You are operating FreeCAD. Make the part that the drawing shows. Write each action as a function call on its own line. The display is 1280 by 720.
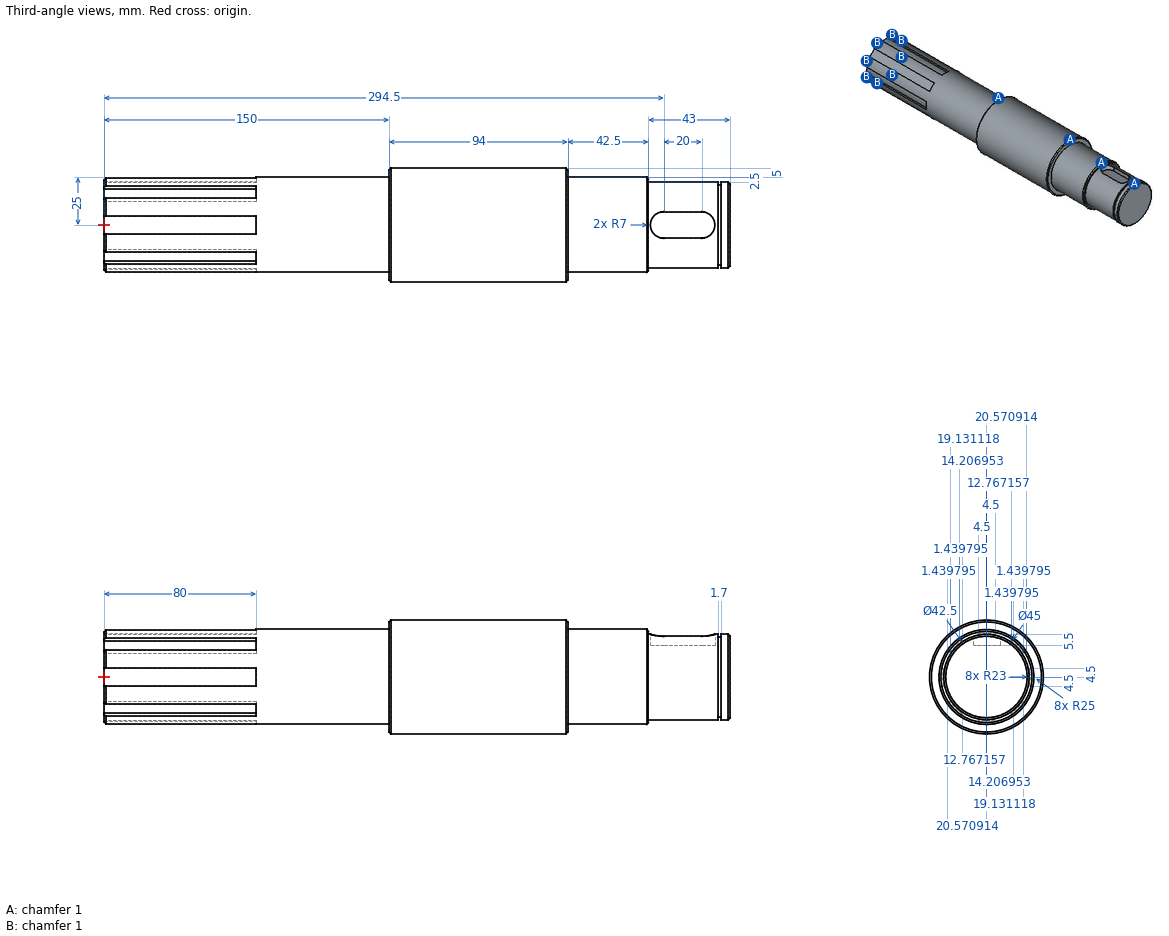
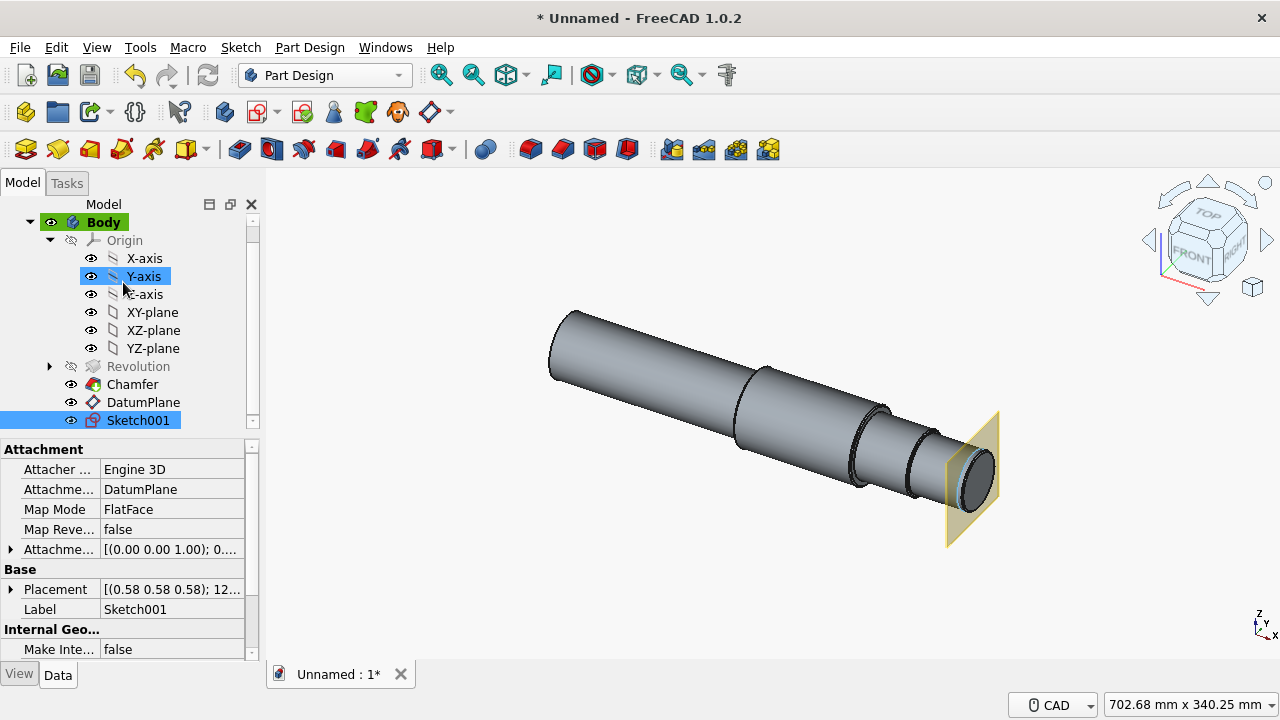
click(240, 150)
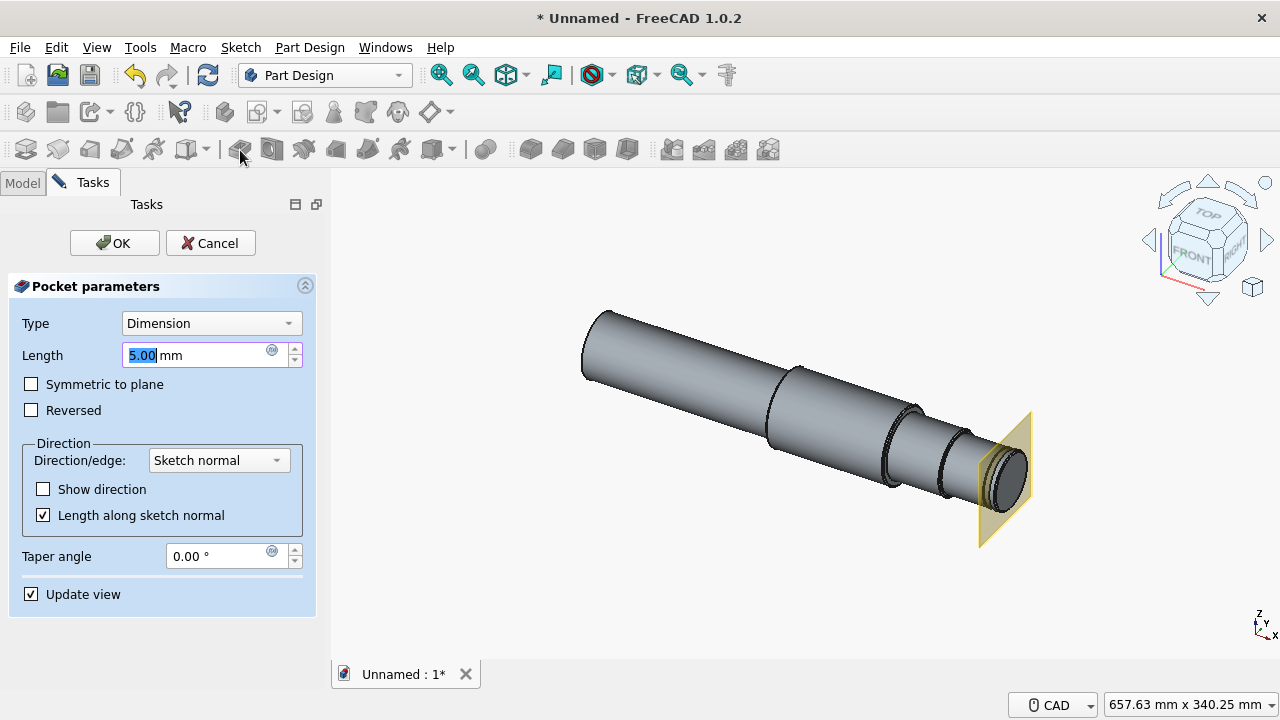
text(1.7)
key(Tab)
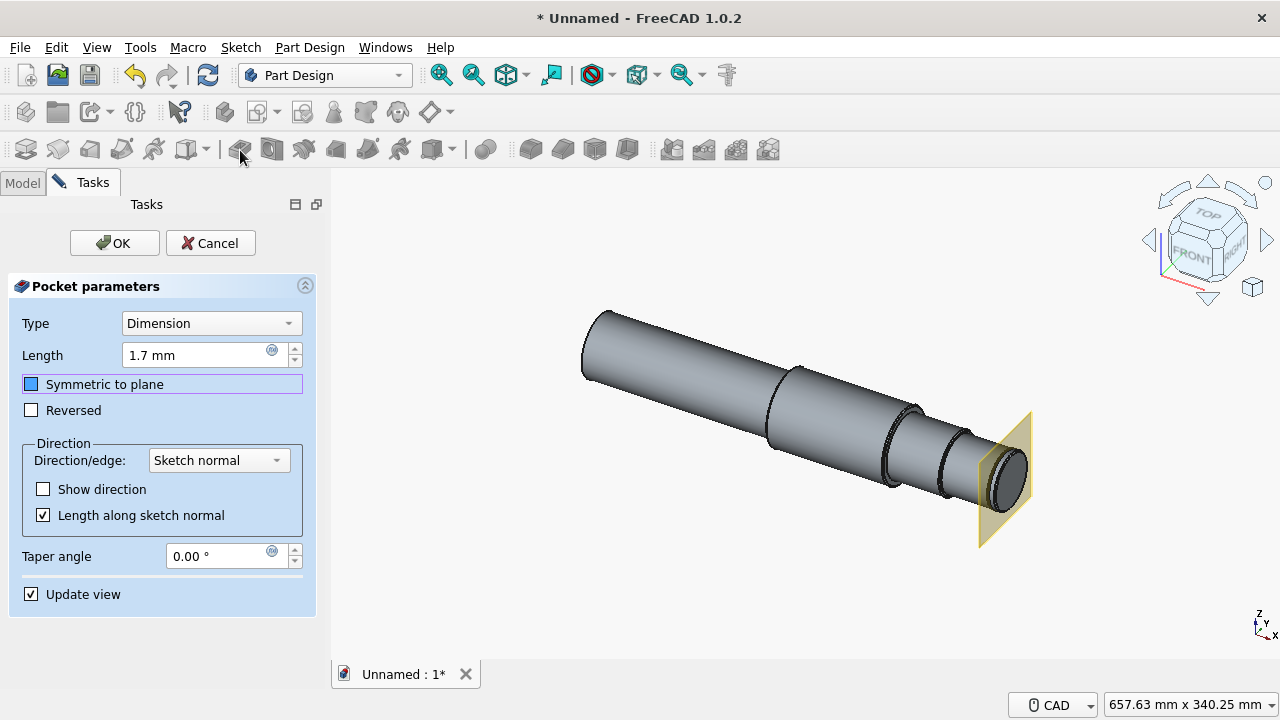
click(115, 243)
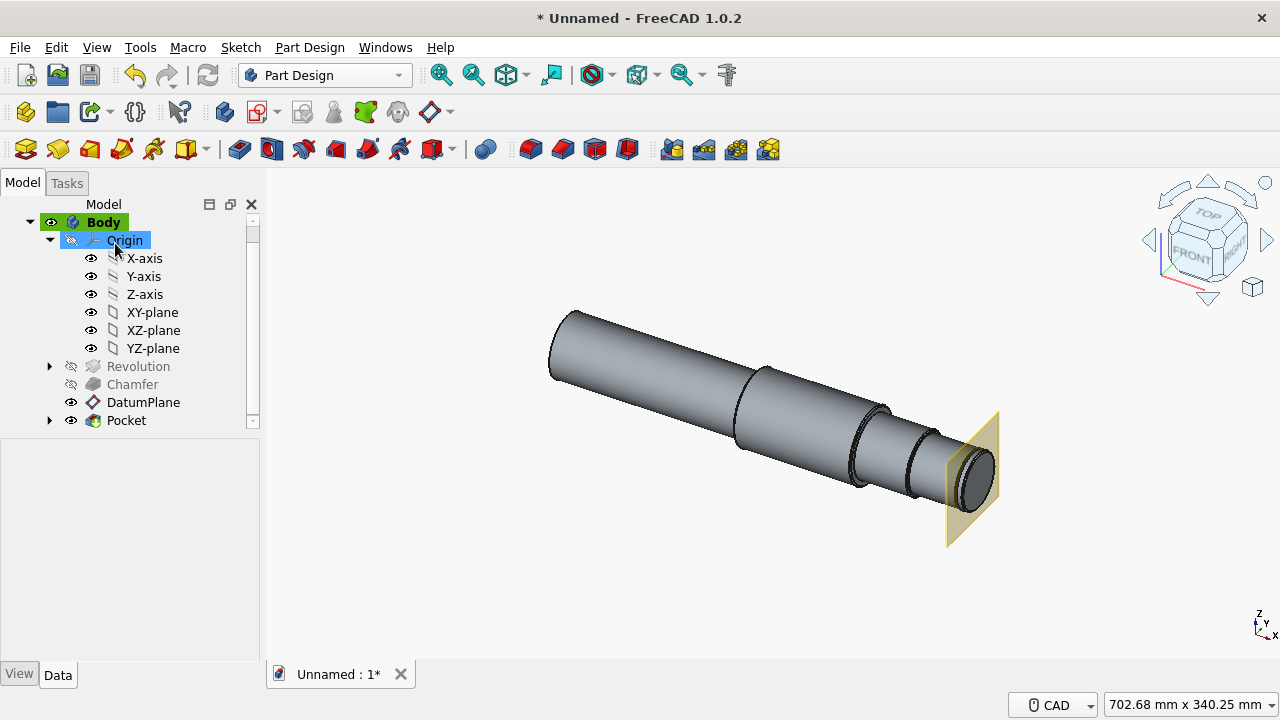
click(116, 402)
key(space)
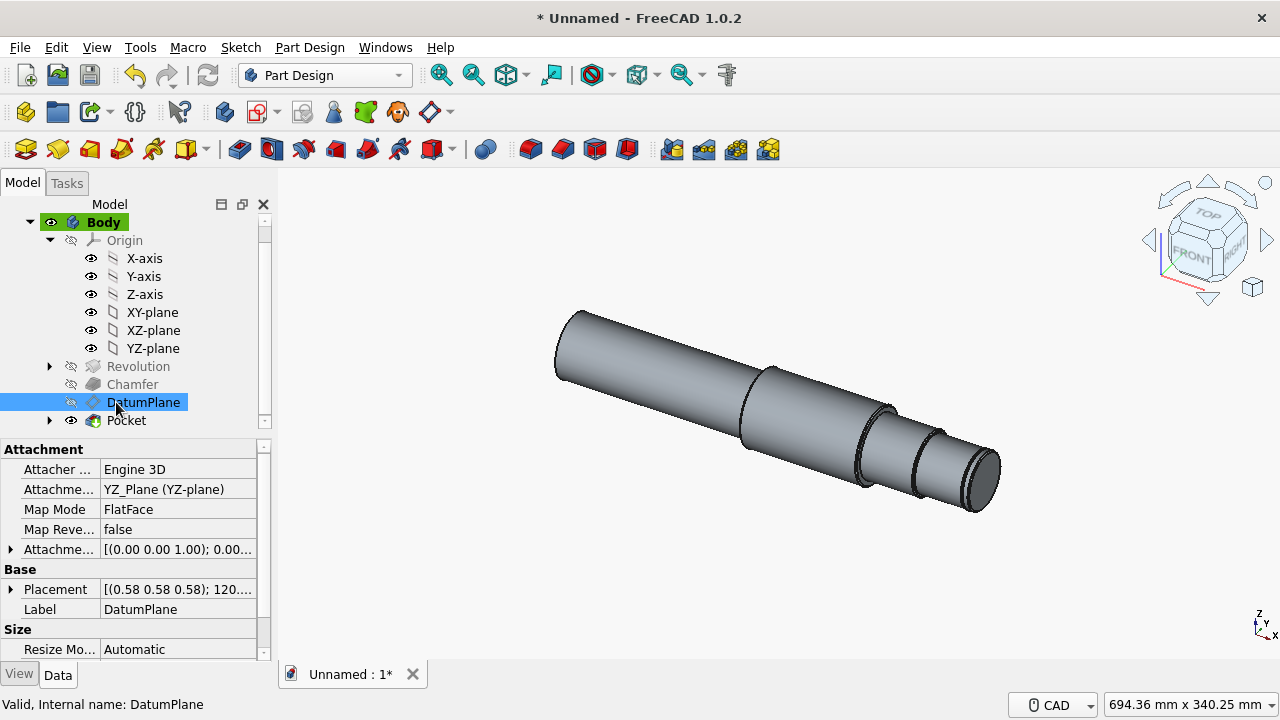
click(136, 312)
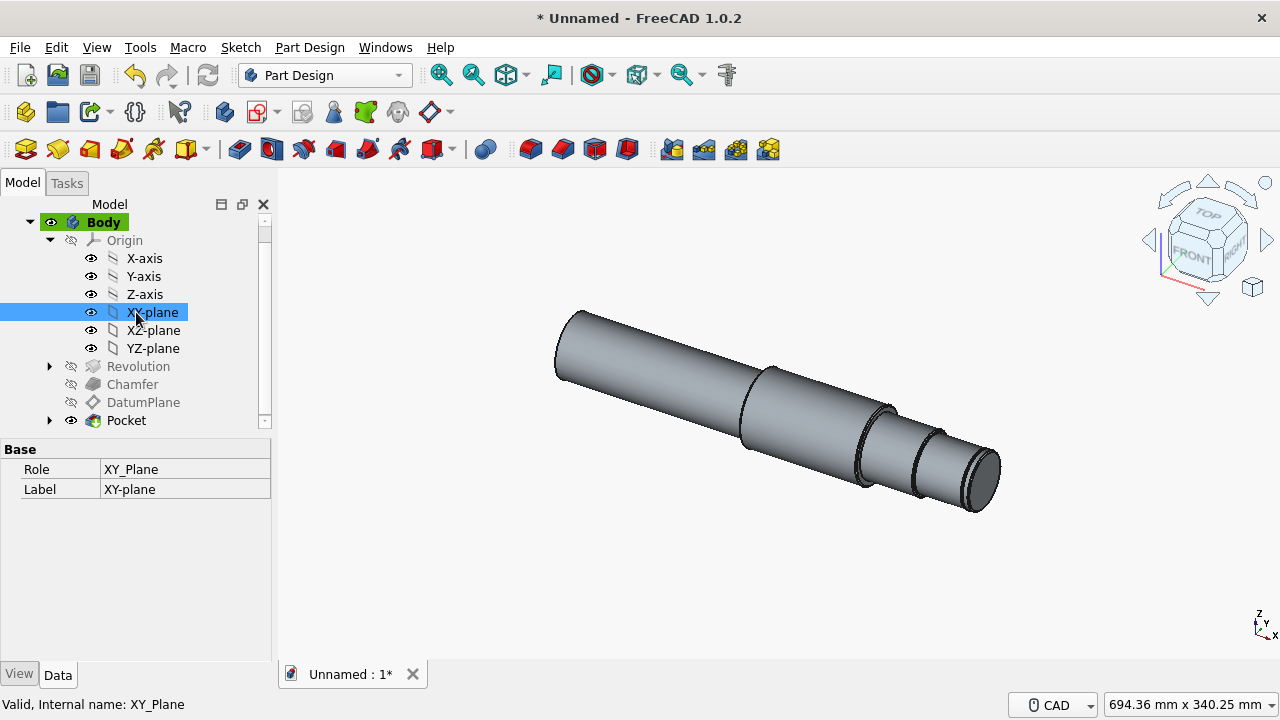
click(430, 112)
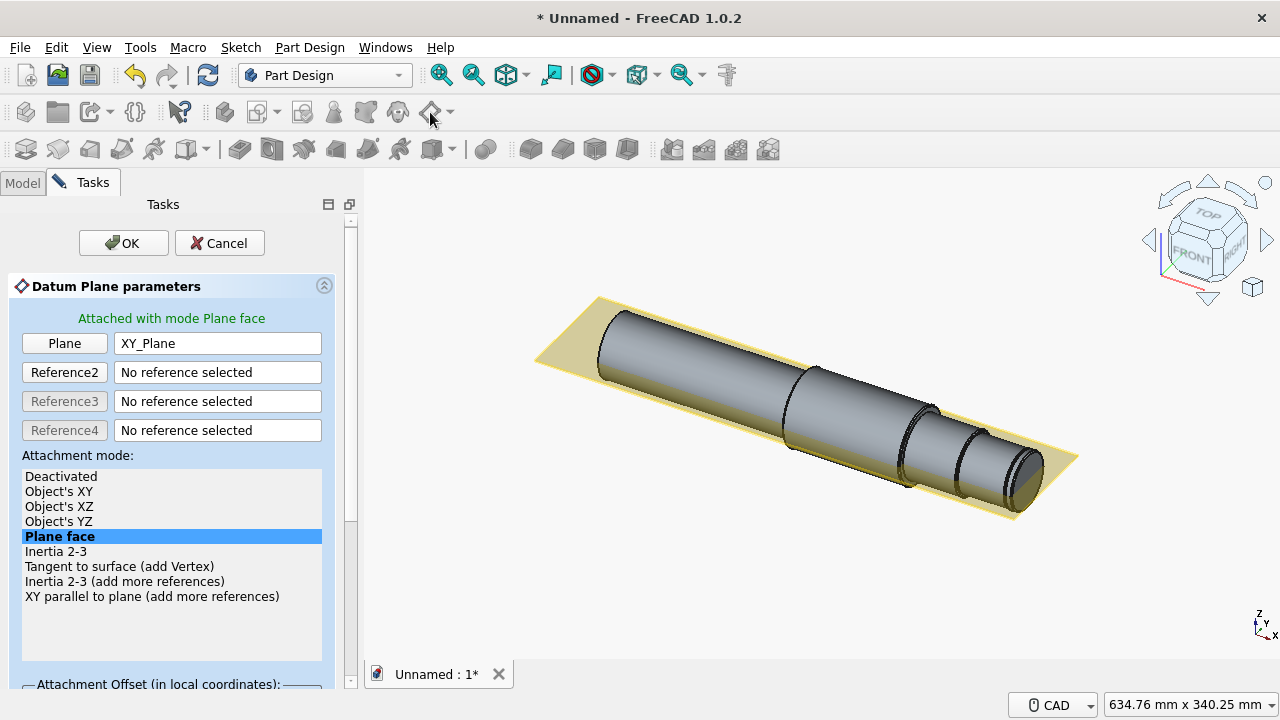
scroll(351, 451, down, 3)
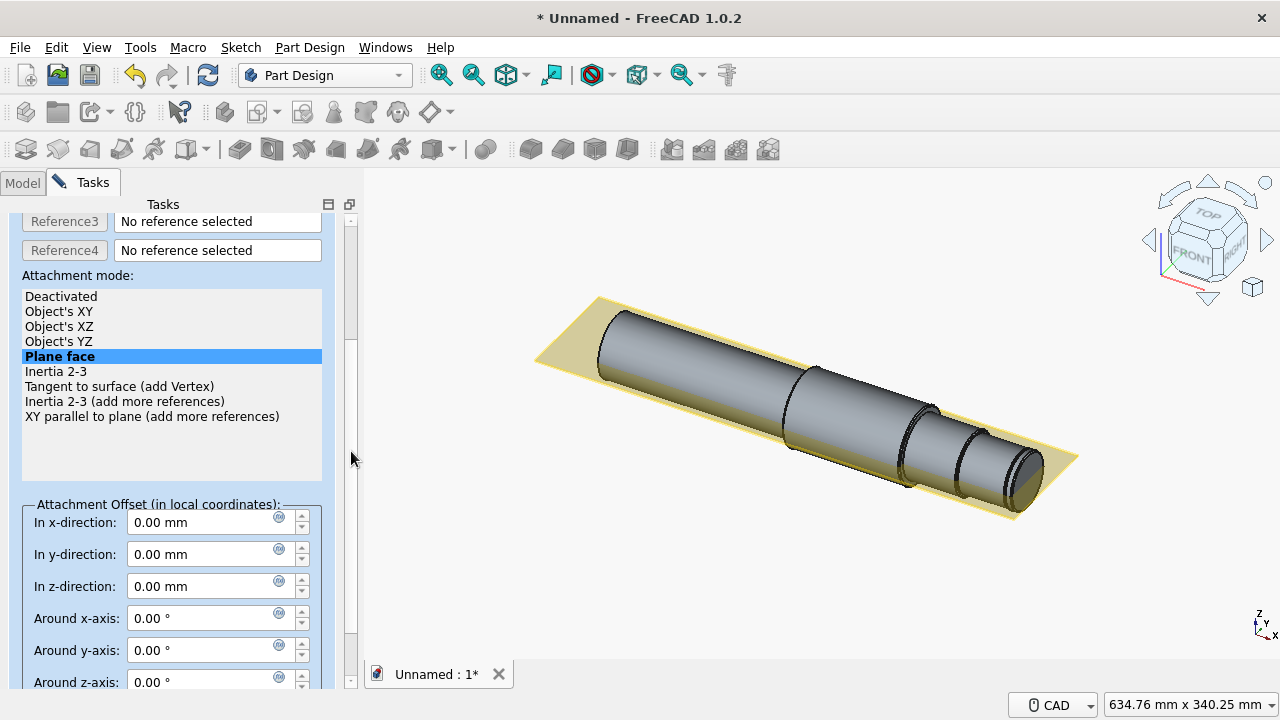
triple_click(210, 586)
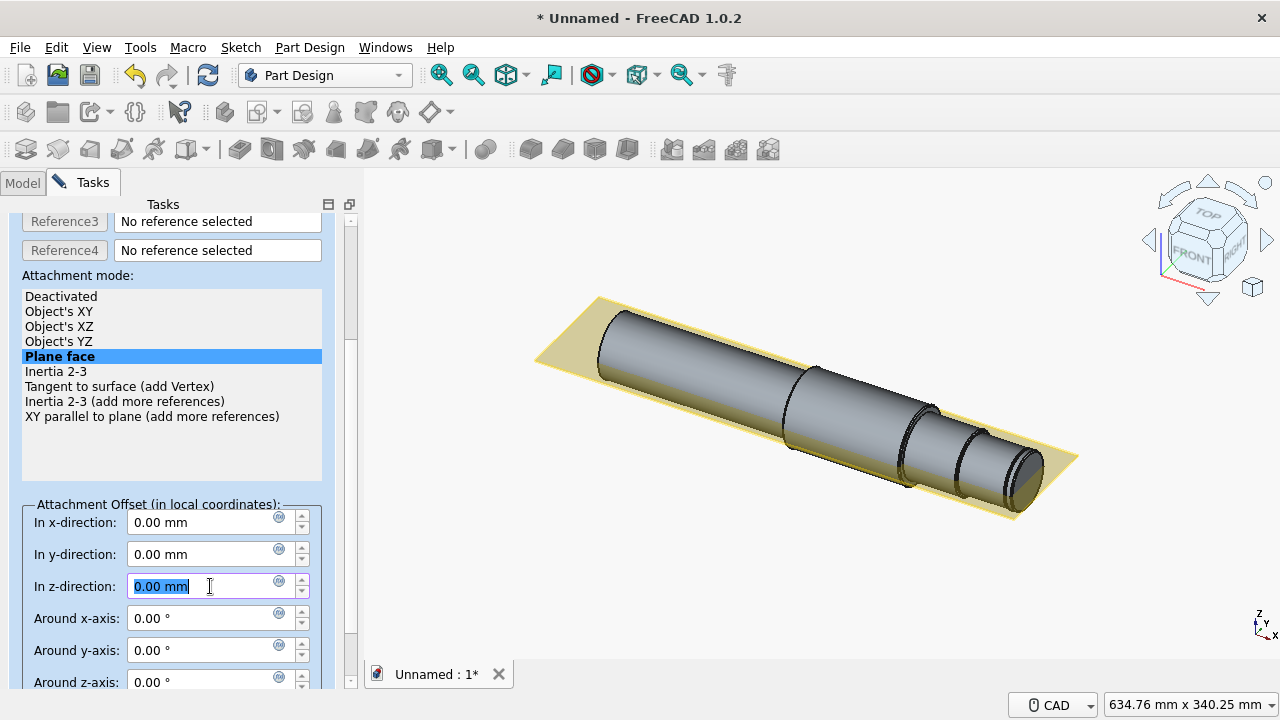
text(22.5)
key(Tab)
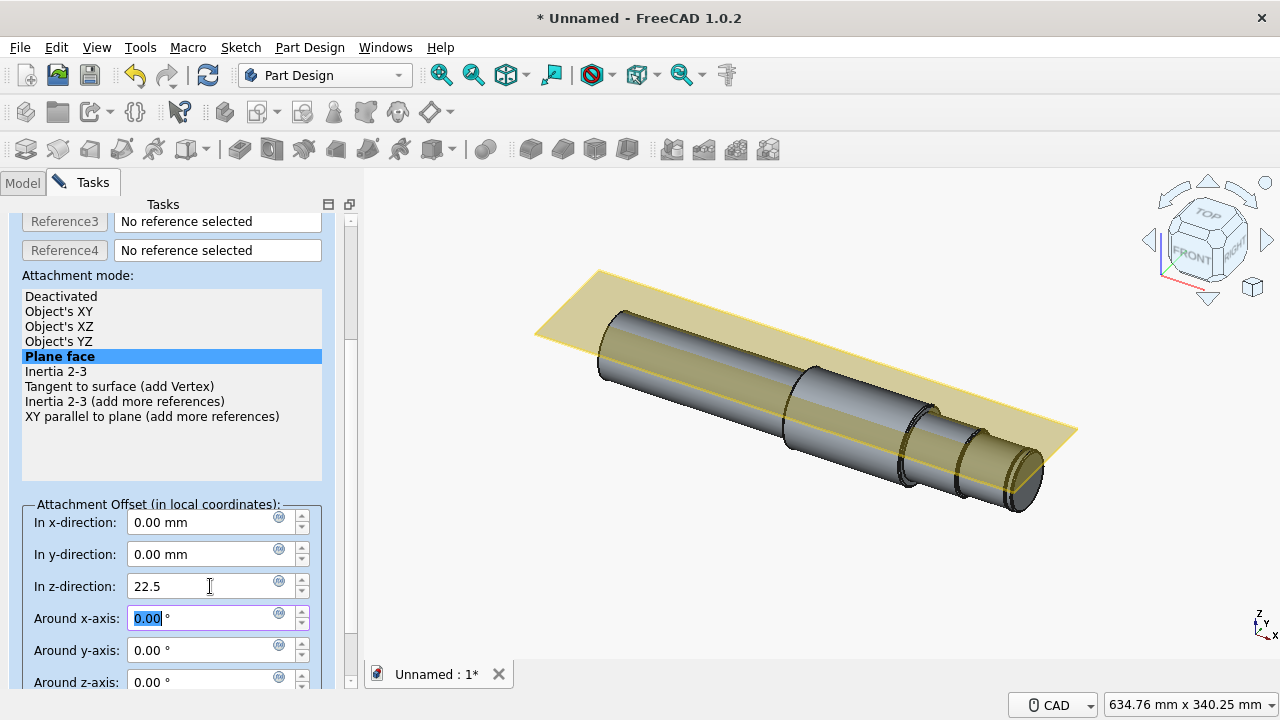
scroll(351, 451, up, 4)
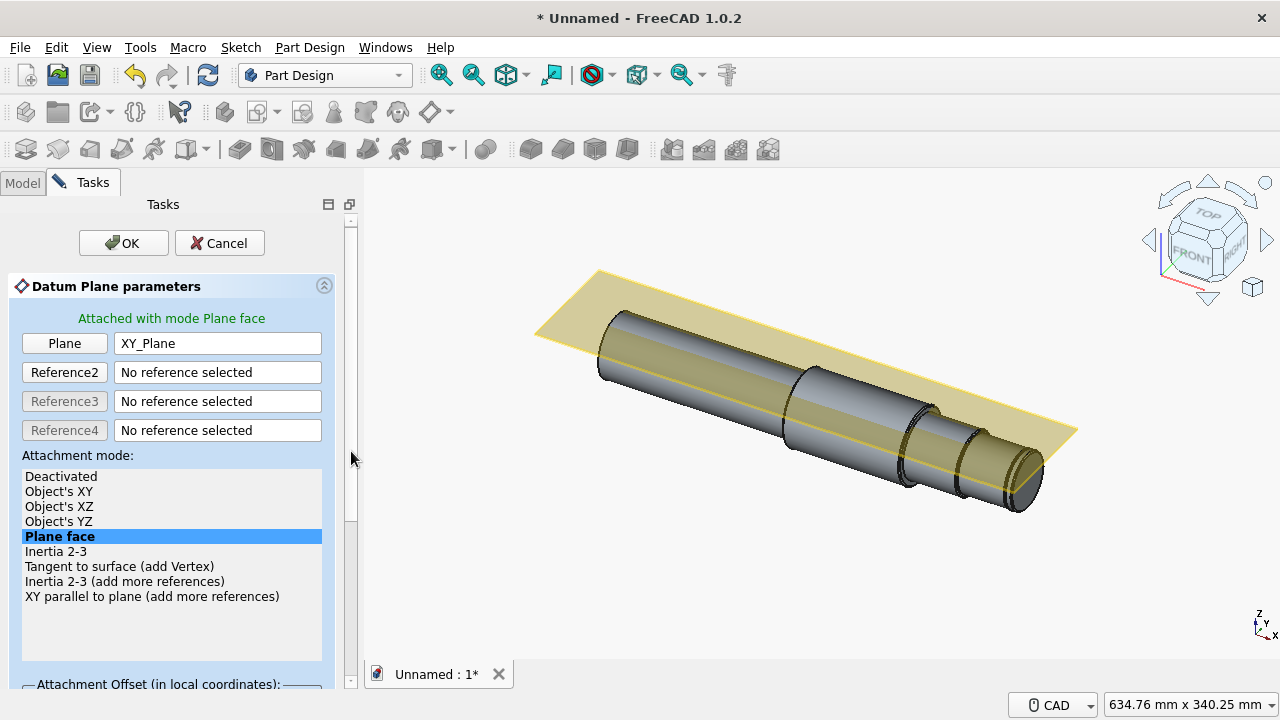
click(124, 243)